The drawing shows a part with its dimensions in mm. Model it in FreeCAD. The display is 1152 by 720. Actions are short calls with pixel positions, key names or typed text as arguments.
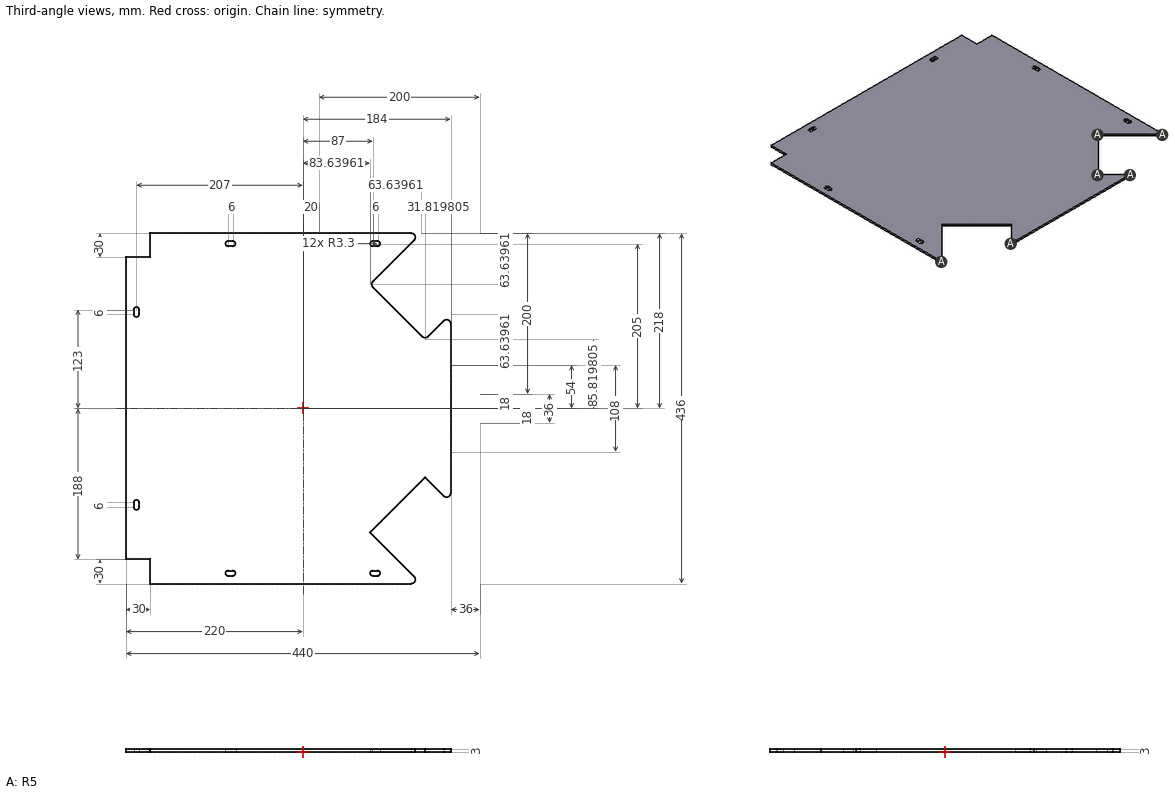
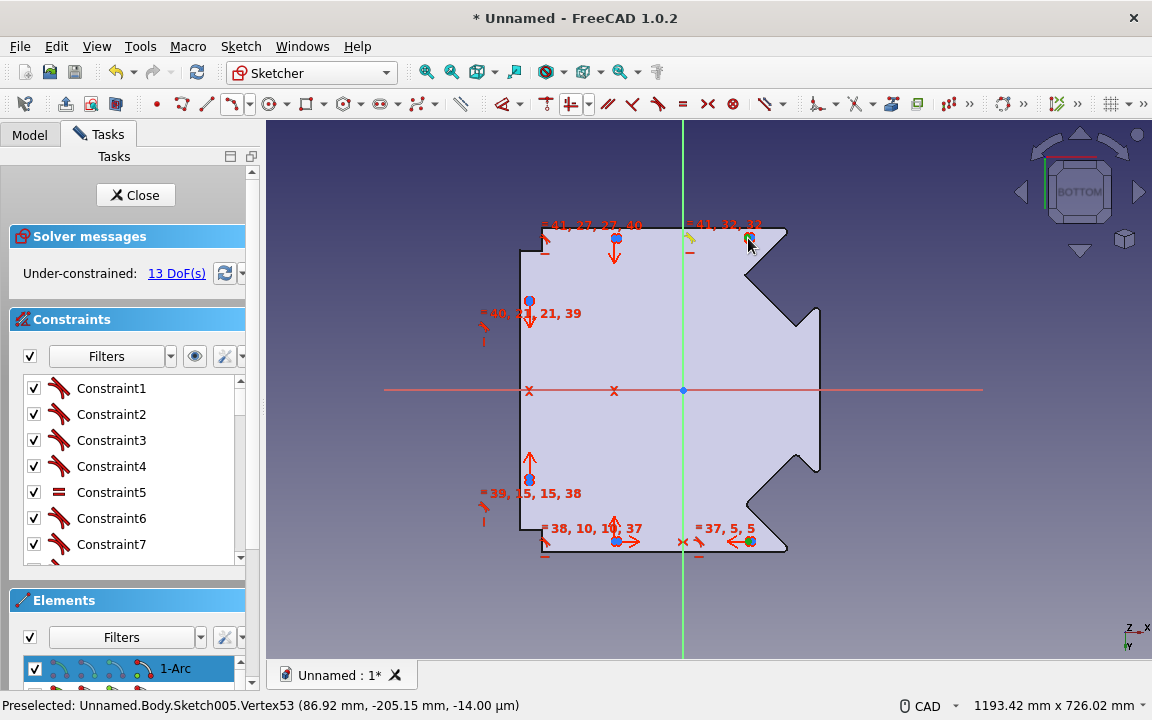
click(393, 390)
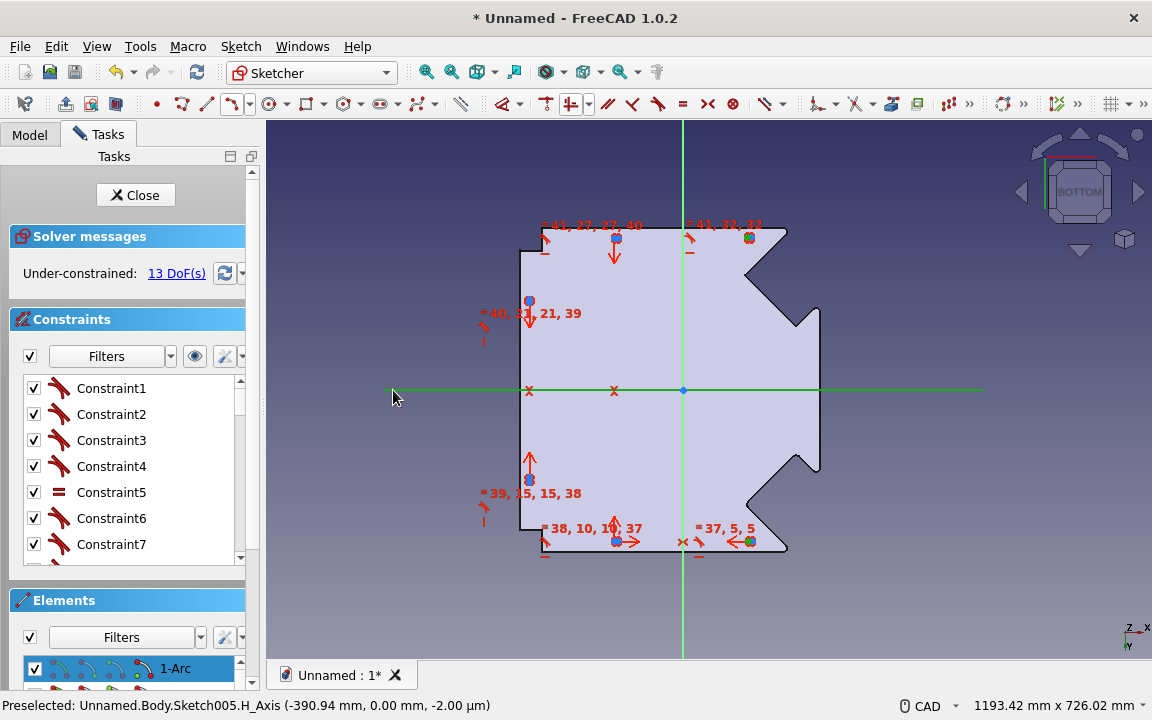
click(708, 104)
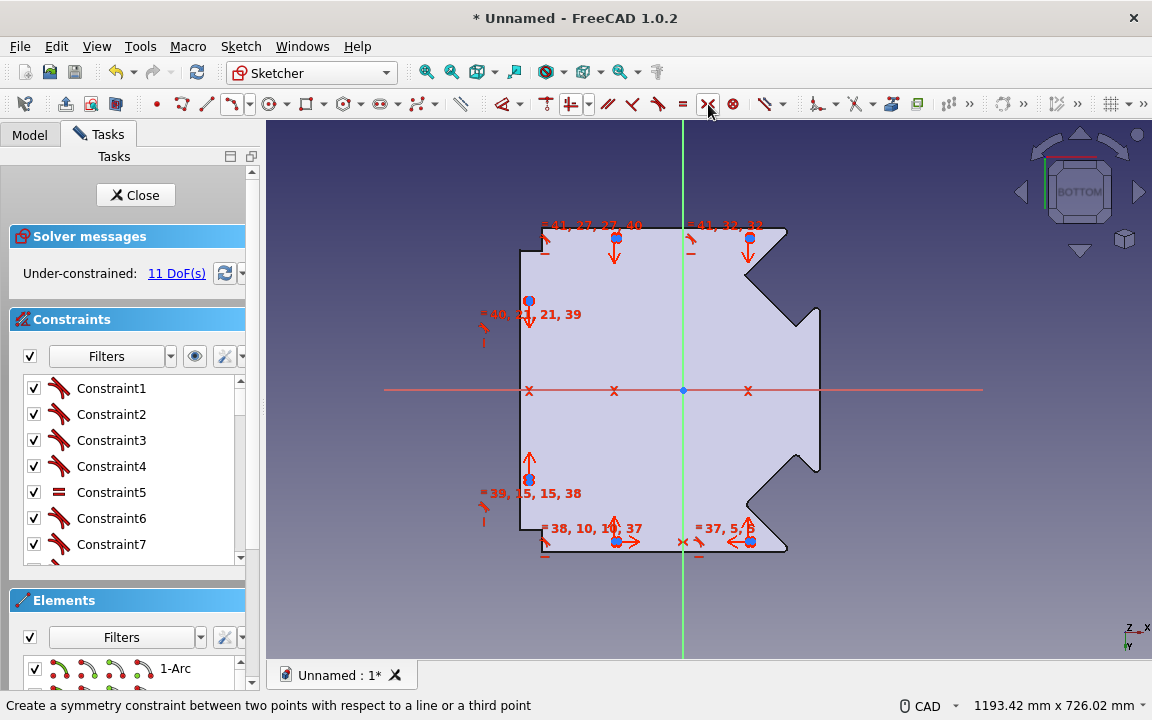
click(502, 104)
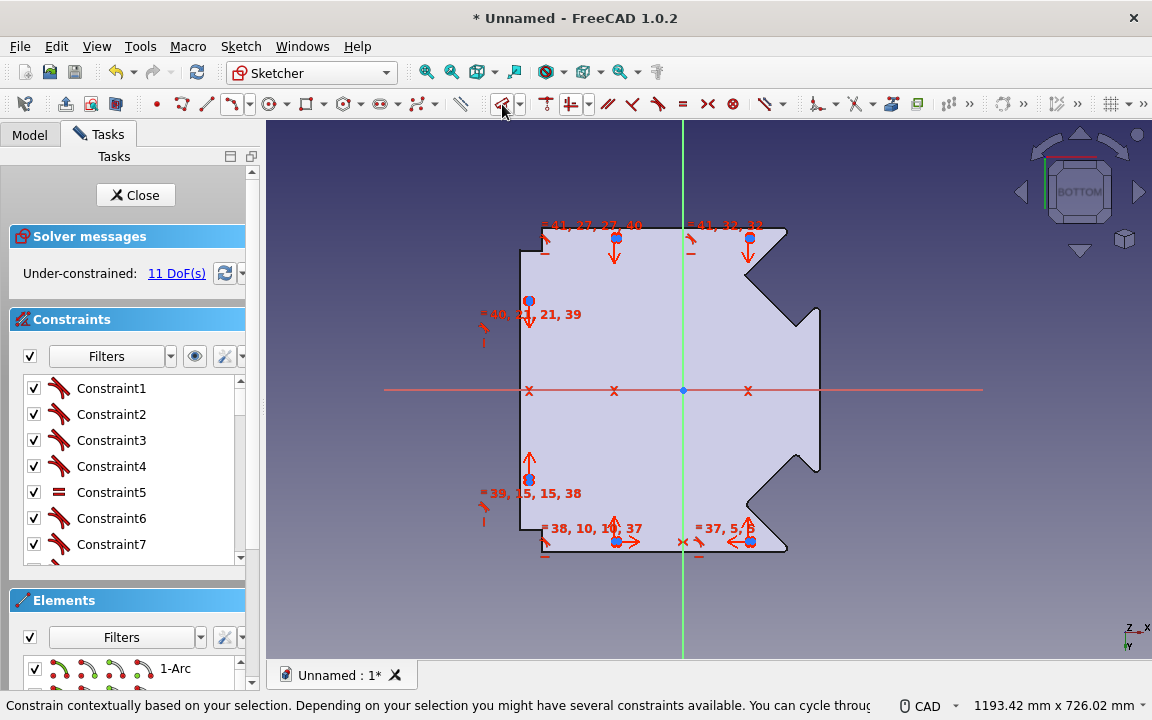
scroll(746, 542, up, 14)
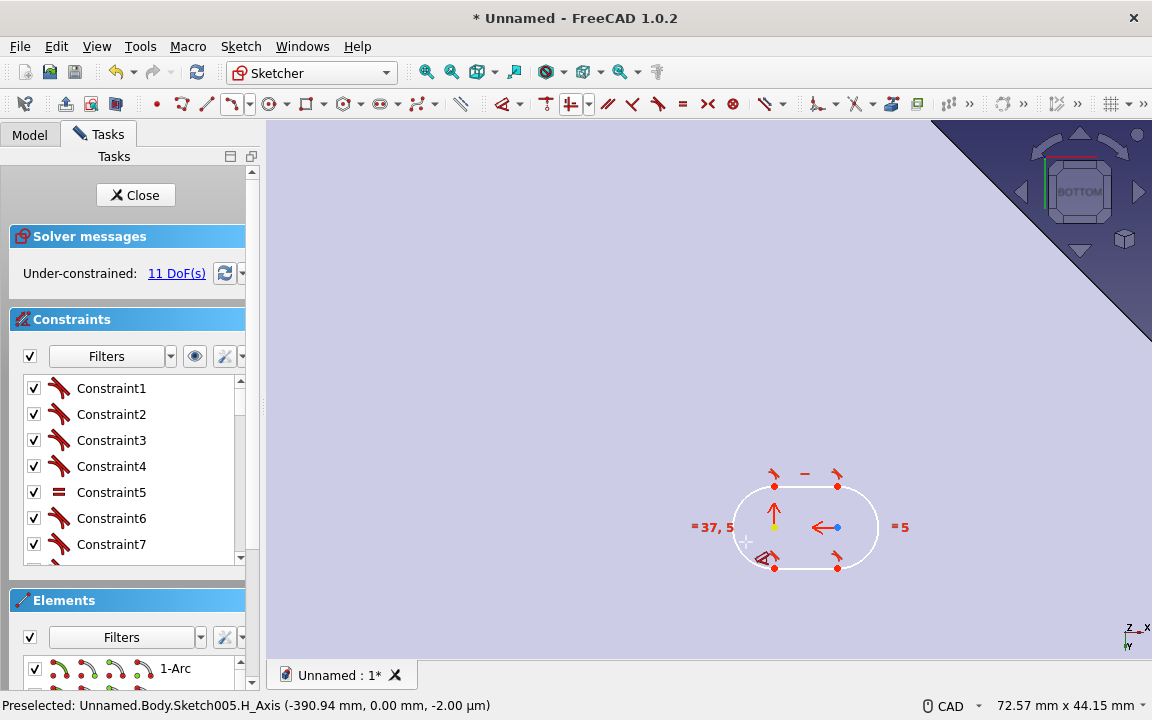
click(733, 528)
click(701, 528)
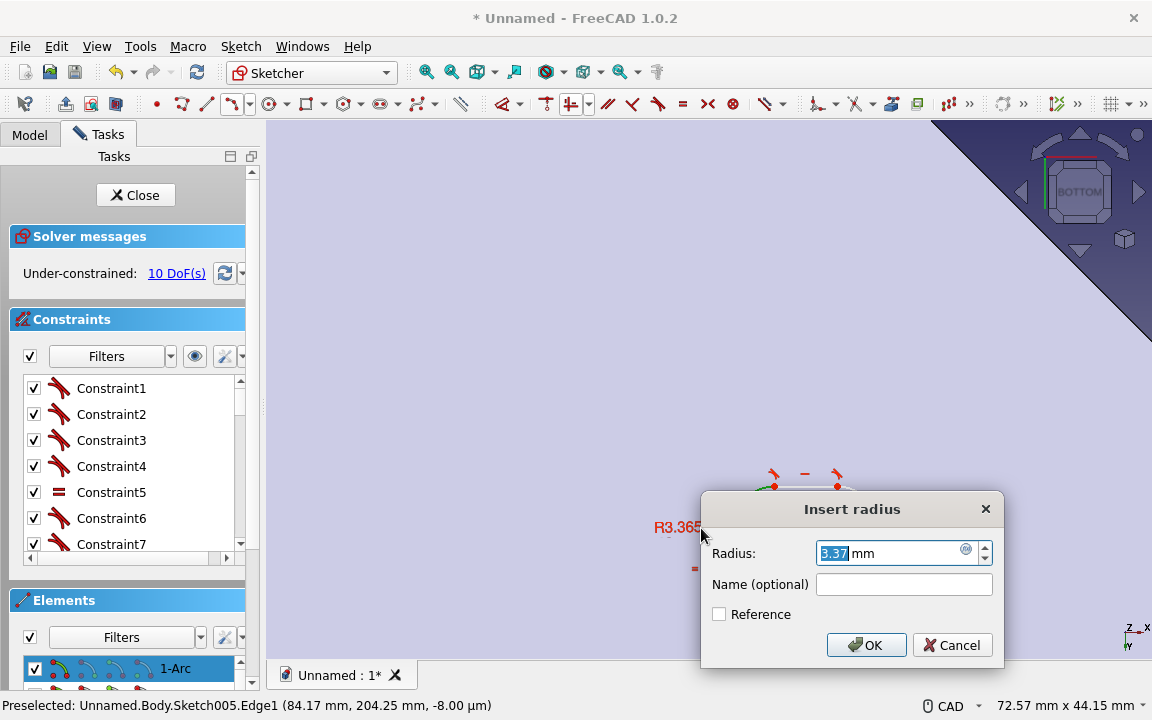
text(3.3)
key(Return)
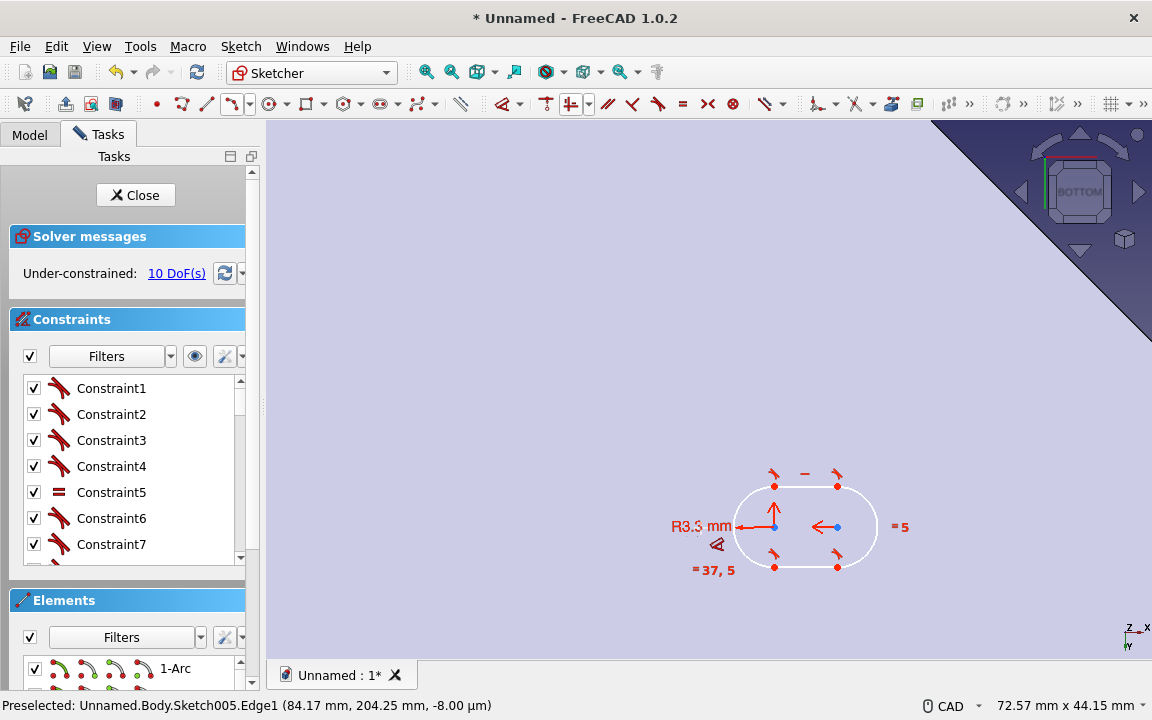
click(793, 487)
click(806, 521)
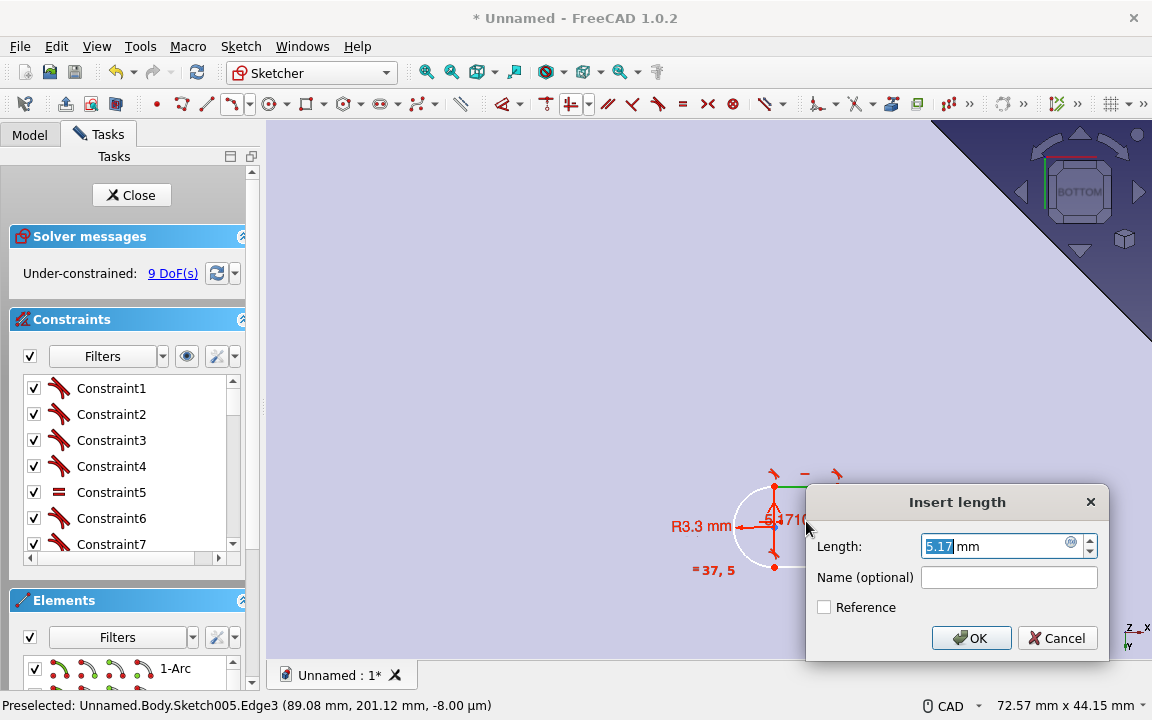
text(6)
key(Return)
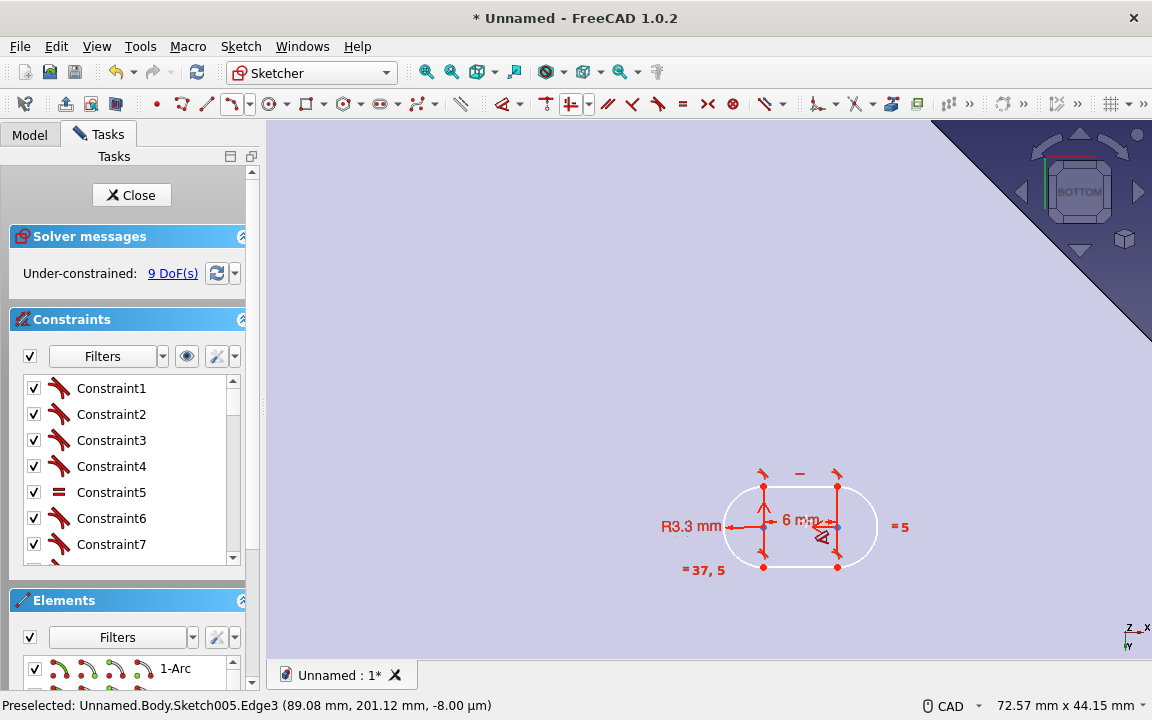
scroll(746, 542, down, 14)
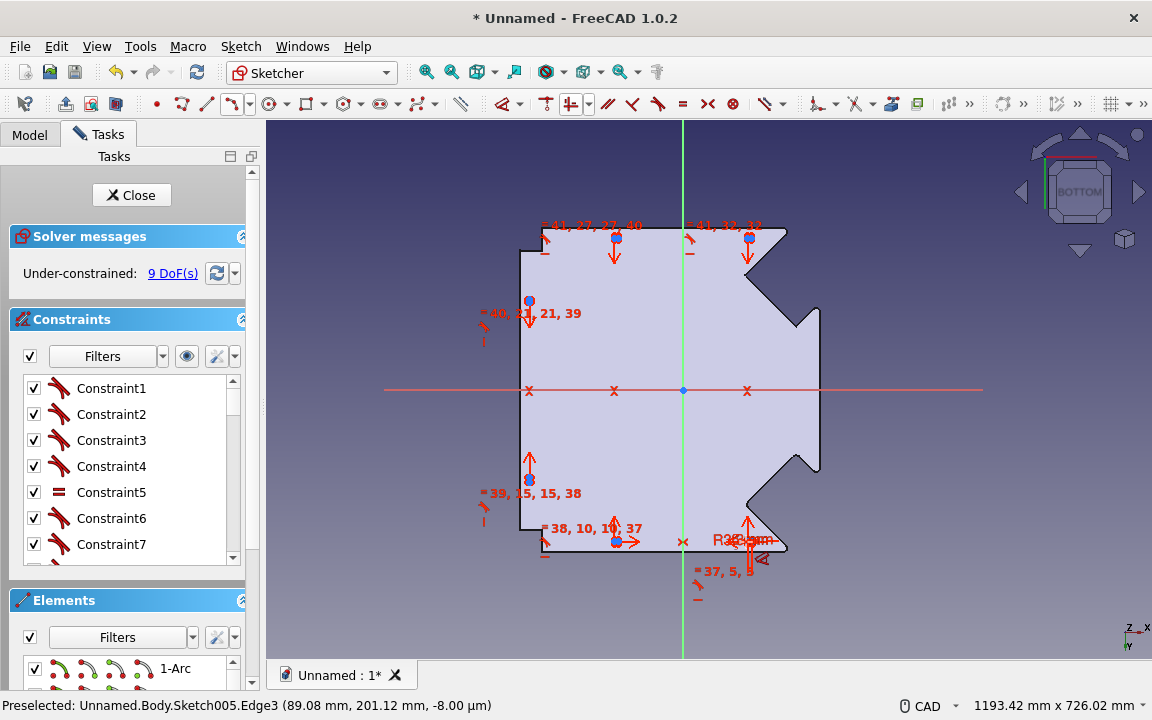
scroll(616, 539, up, 13)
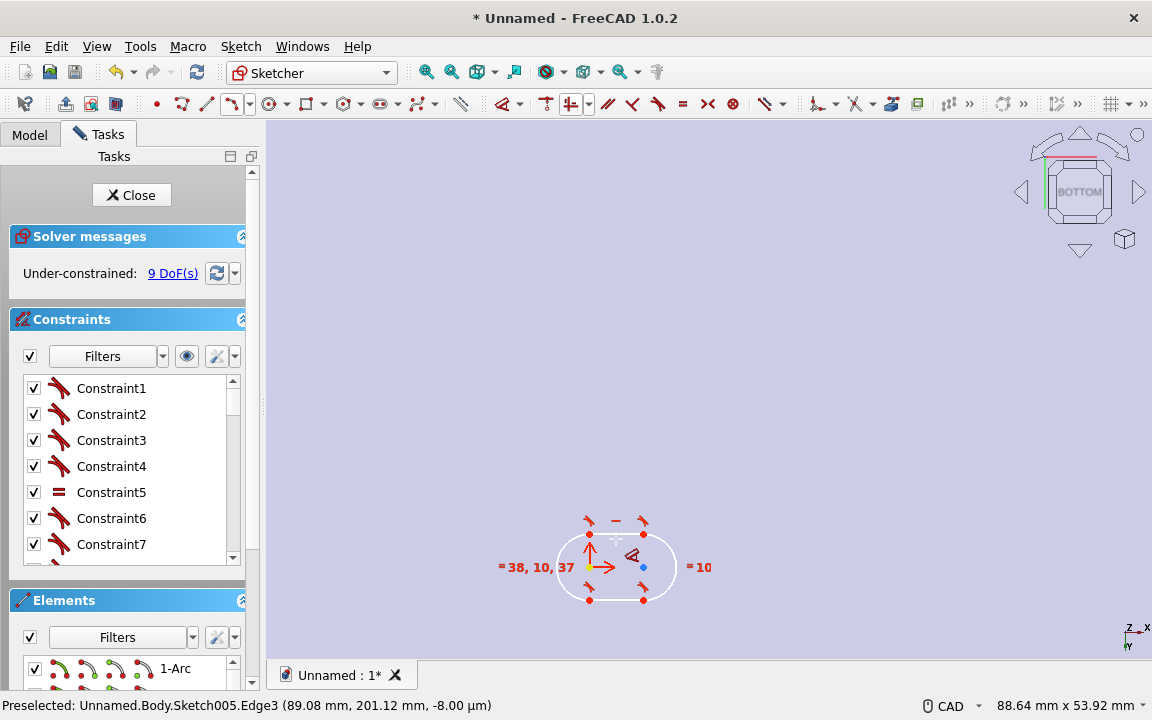
click(606, 534)
click(617, 568)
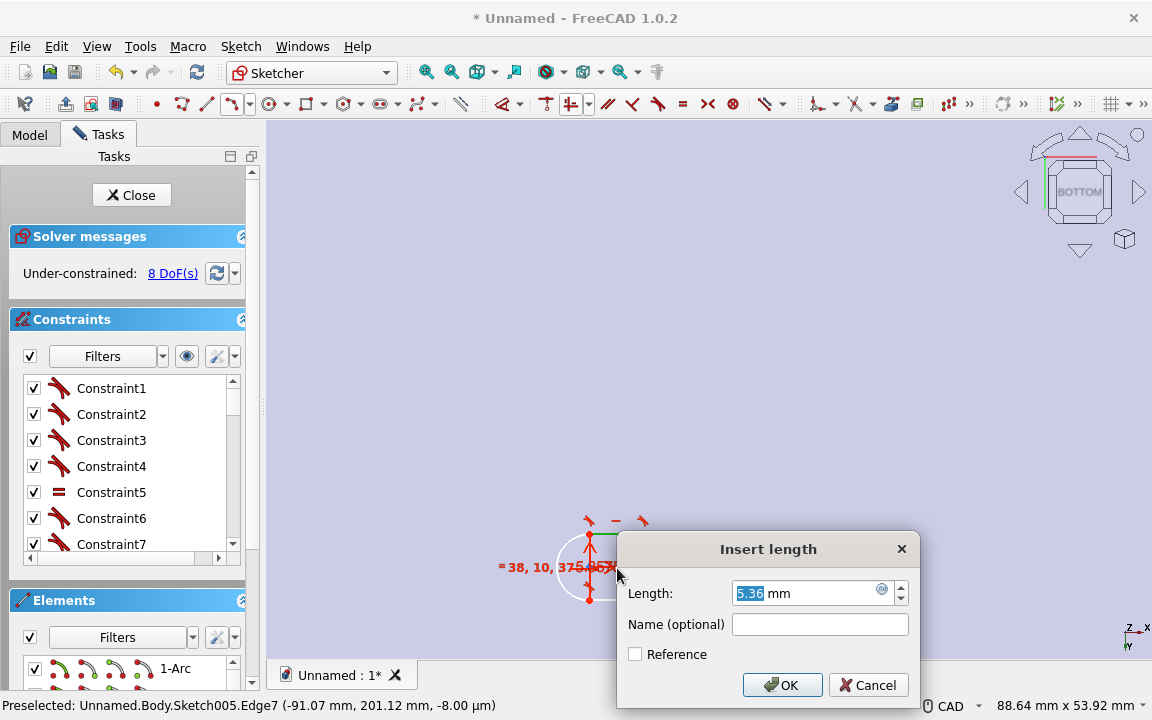
text(6)
key(Return)